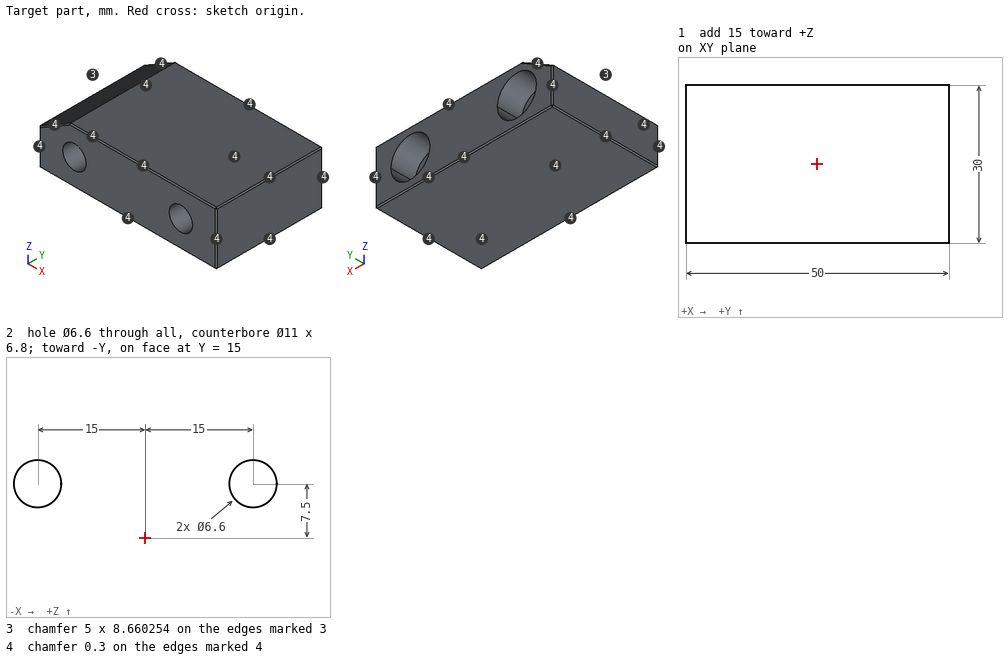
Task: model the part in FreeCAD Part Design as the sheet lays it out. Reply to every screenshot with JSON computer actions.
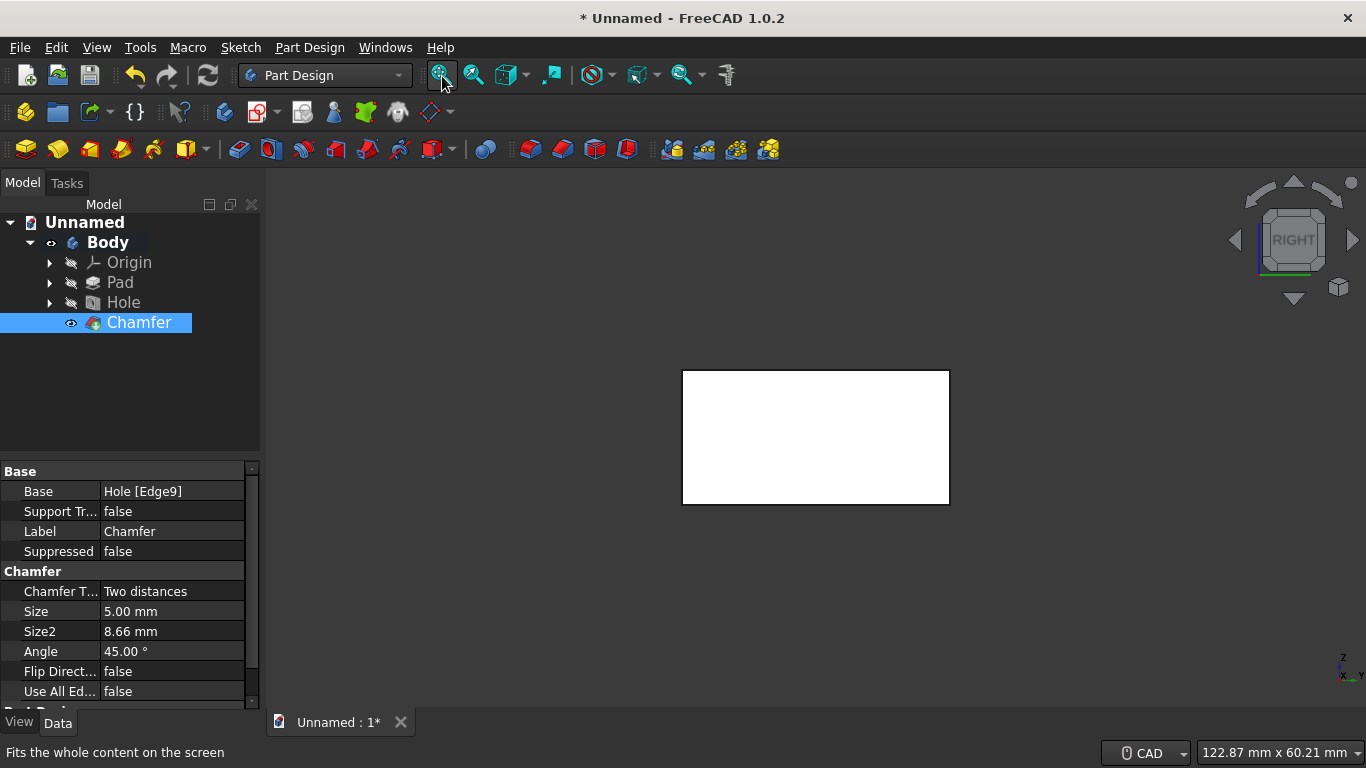
{"action": "key", "text": "5"}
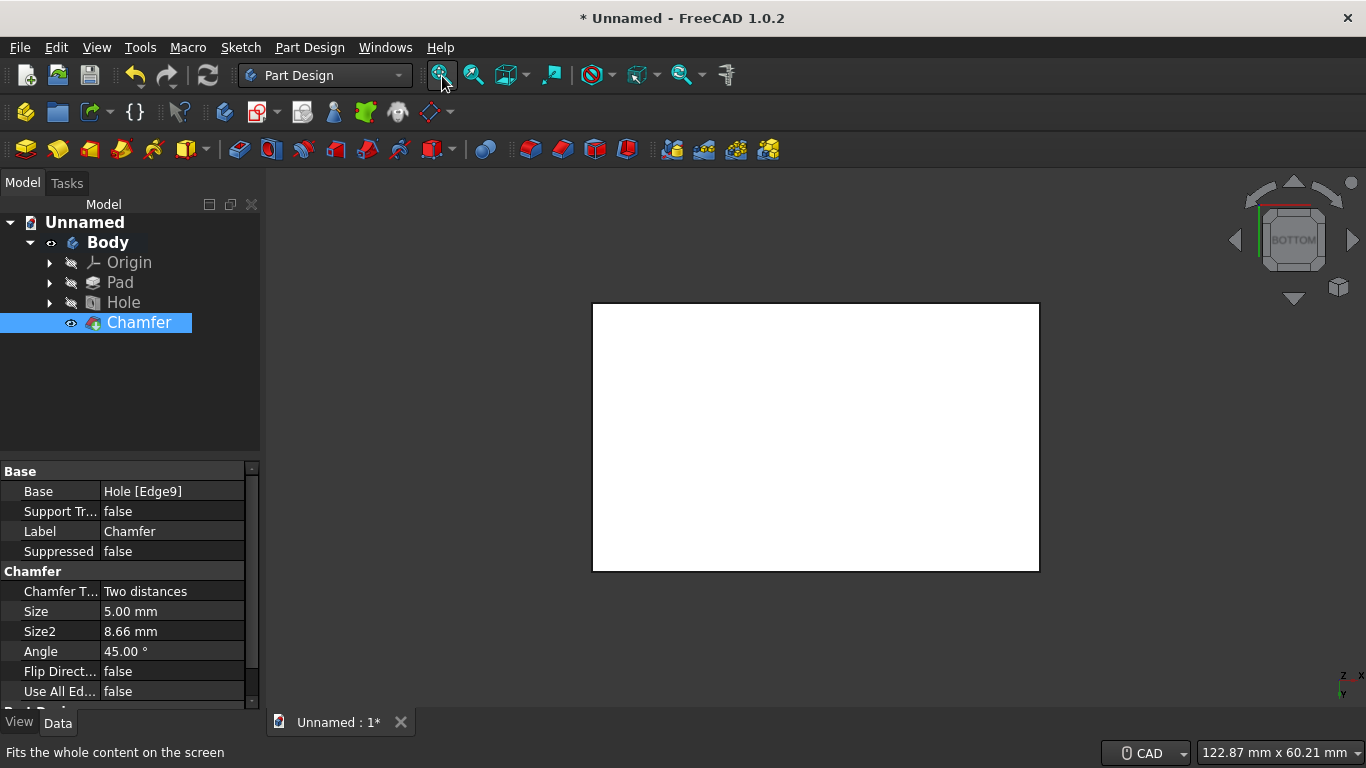
{"action": "left_click", "coordinate": [880, 436], "text": "ctrl"}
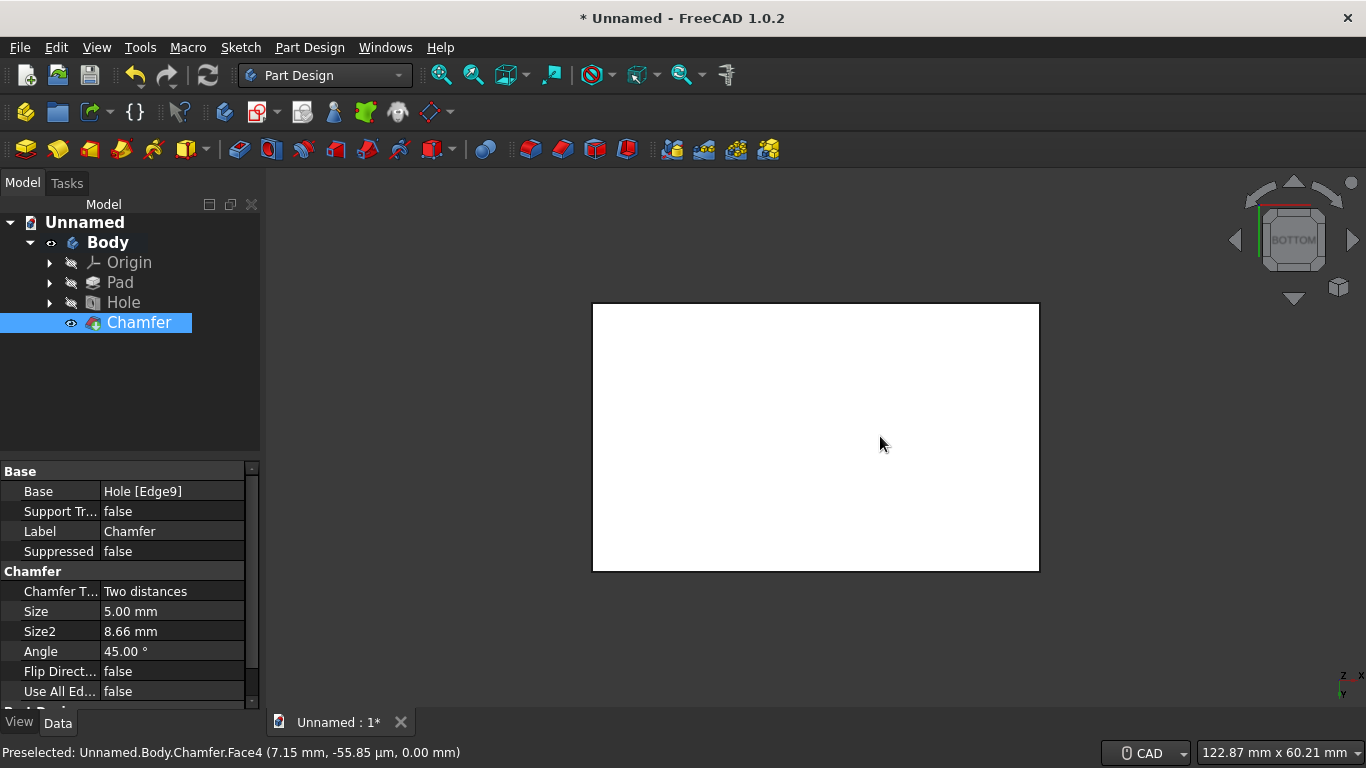
{"action": "key", "text": "4"}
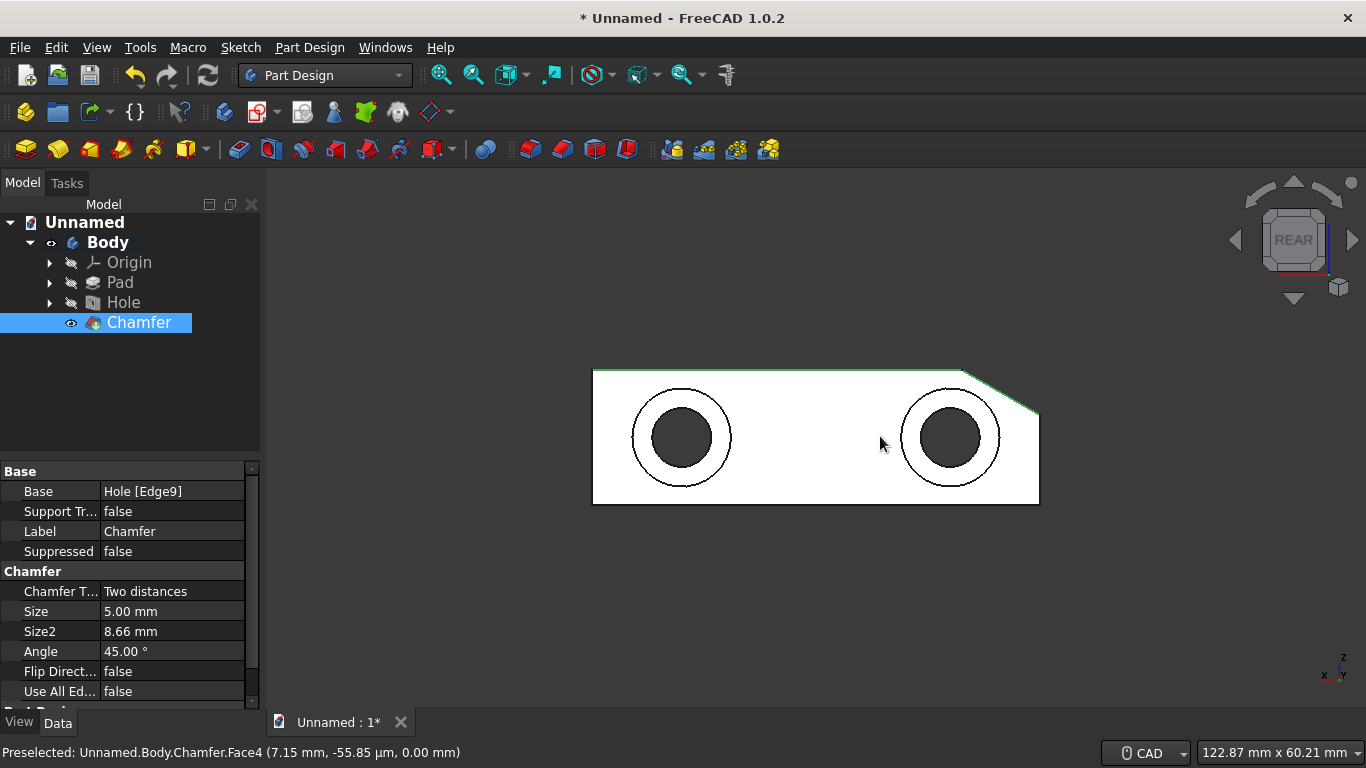
{"action": "left_click", "coordinate": [442, 76]}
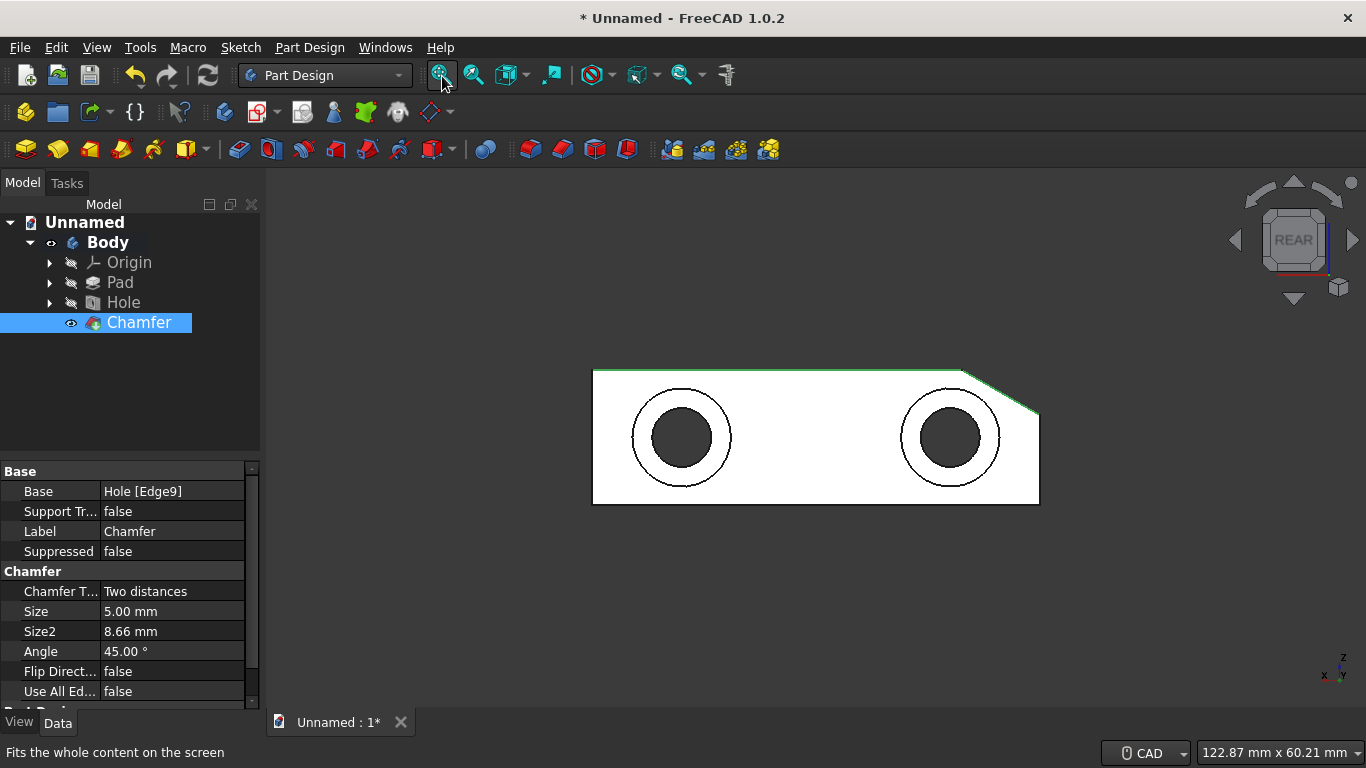
{"action": "left_click", "coordinate": [1040, 459], "text": "ctrl"}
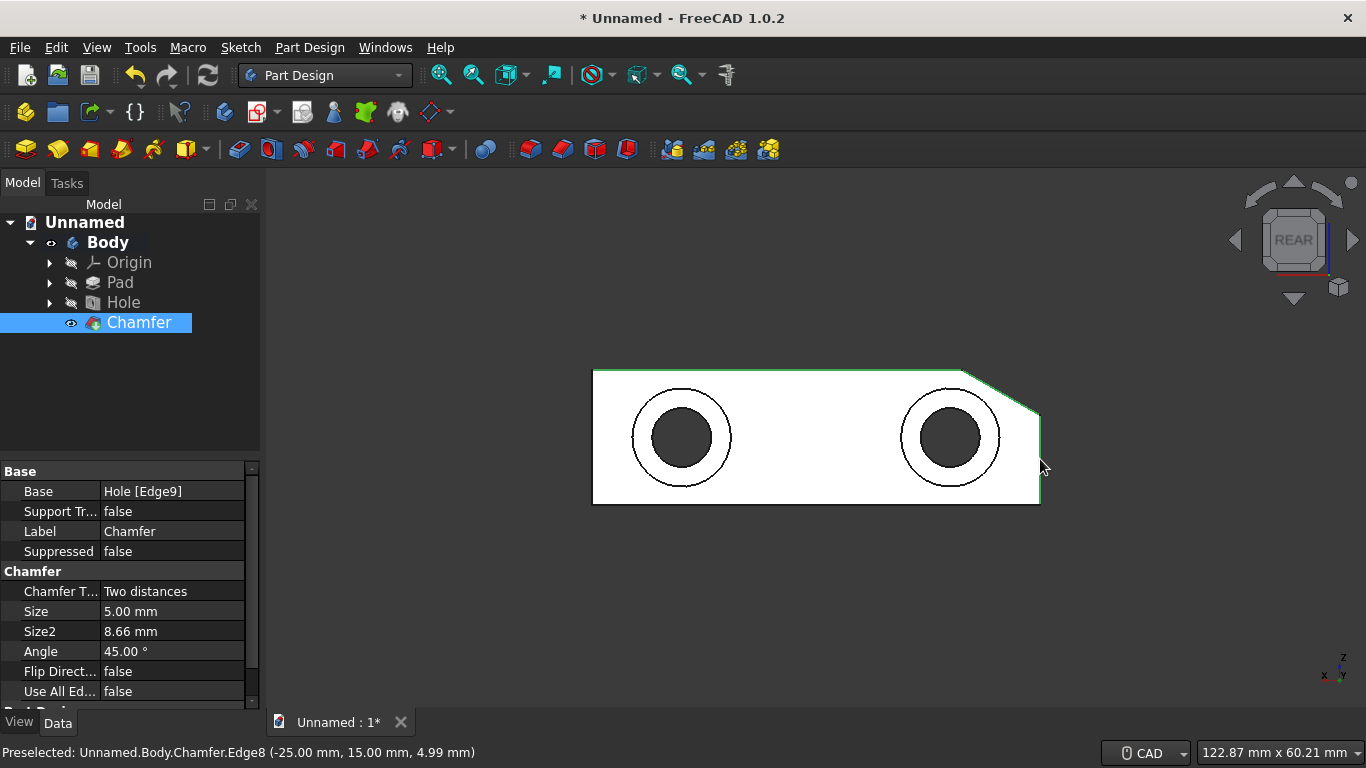
{"action": "left_click", "coordinate": [564, 150]}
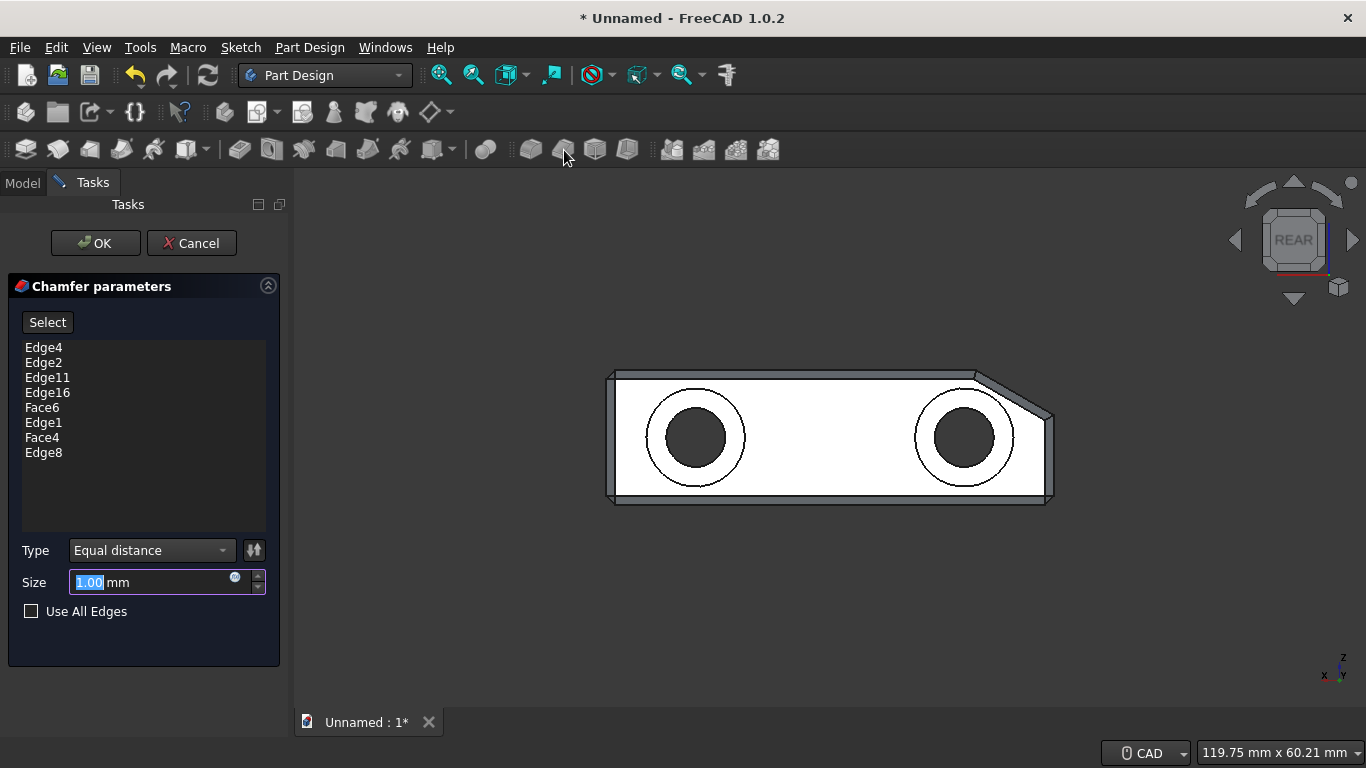
{"action": "type", "text": "0.3"}
{"action": "key", "text": "Tab"}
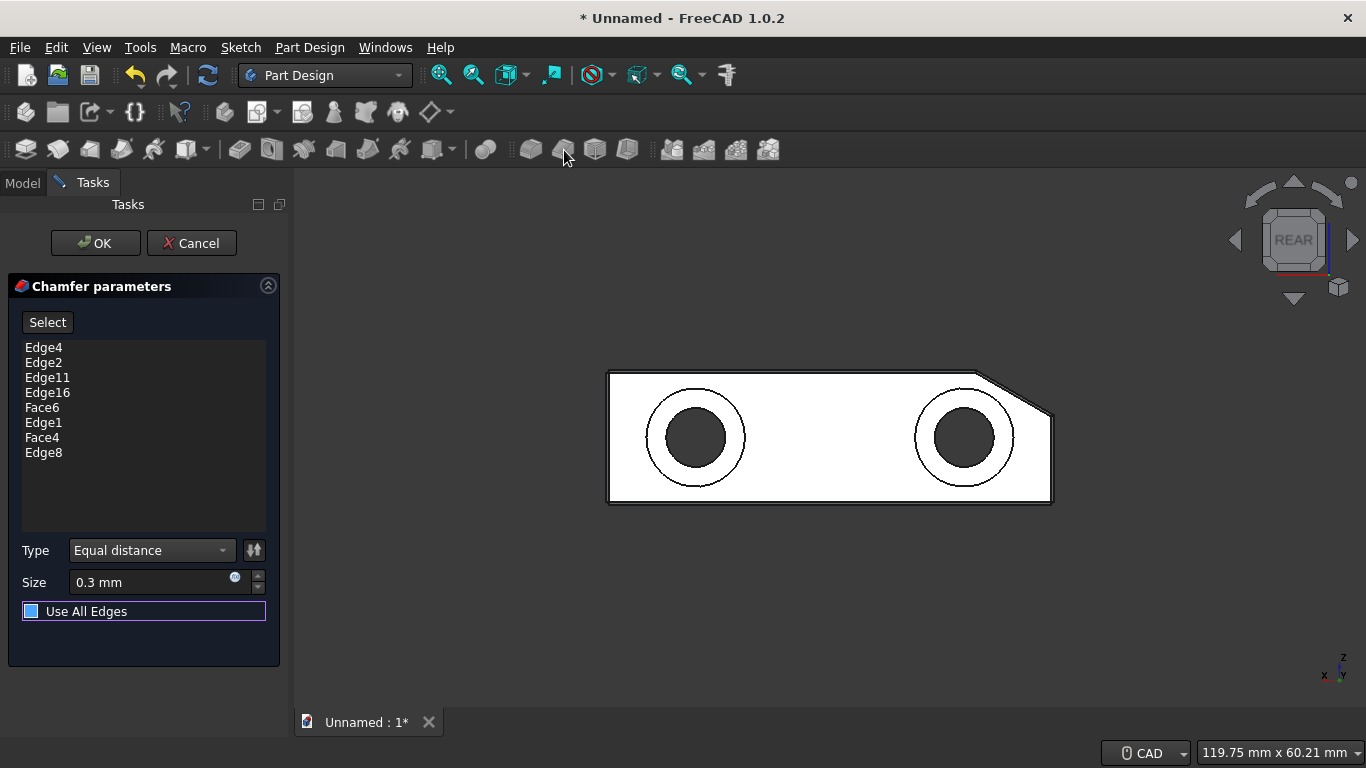
{"action": "left_click", "coordinate": [96, 243]}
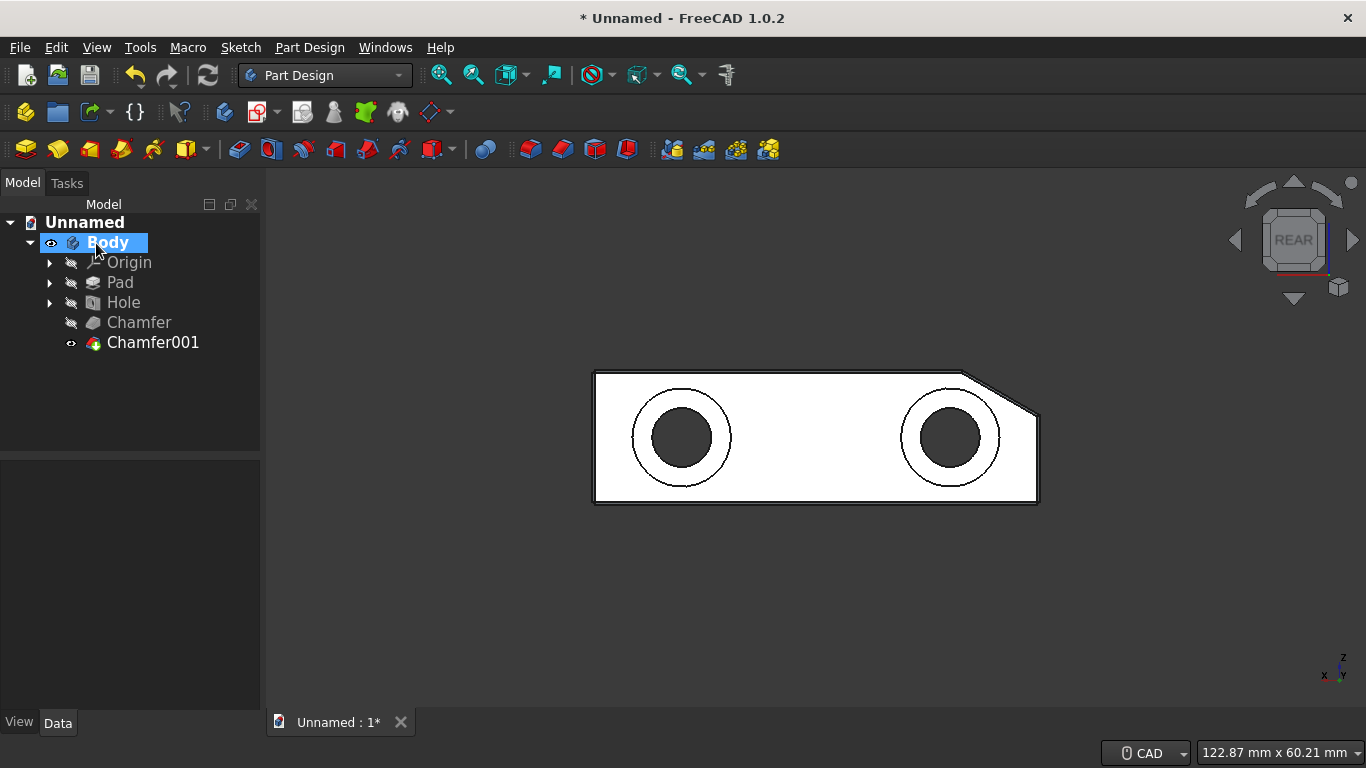
{"action": "key", "text": "0"}